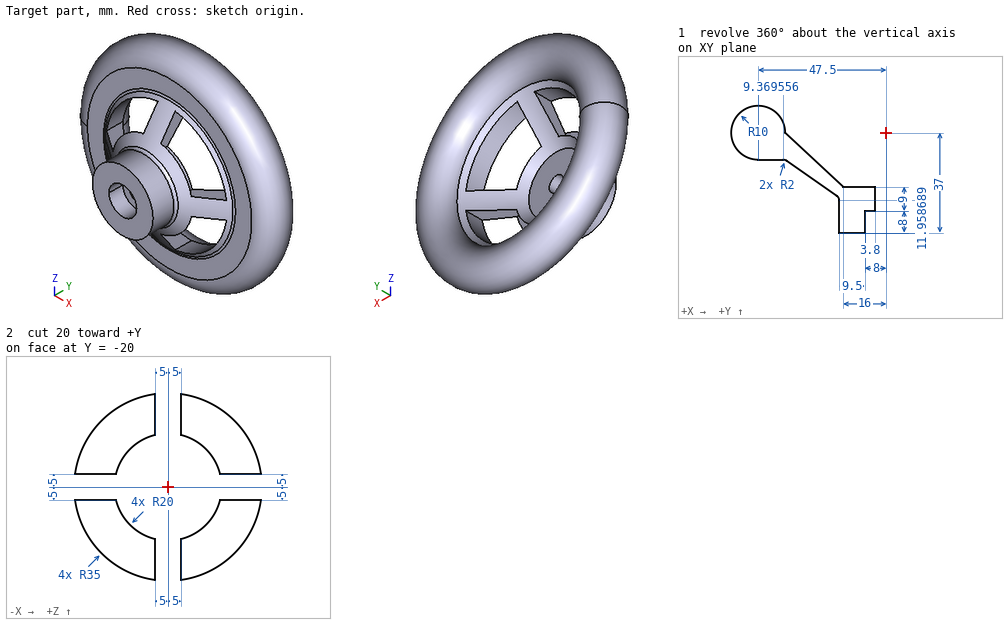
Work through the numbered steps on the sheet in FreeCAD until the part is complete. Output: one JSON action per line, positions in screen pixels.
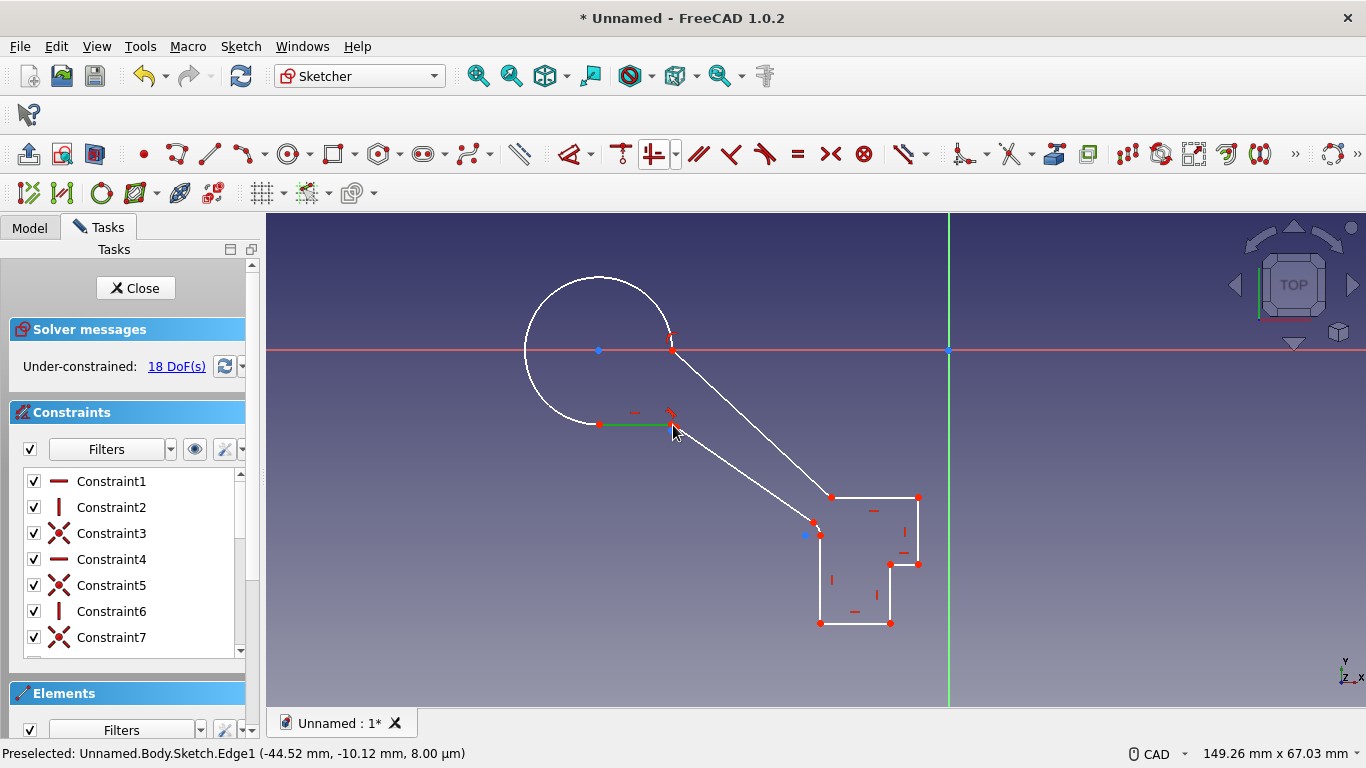
{"action": "left_click", "coordinate": [609, 278]}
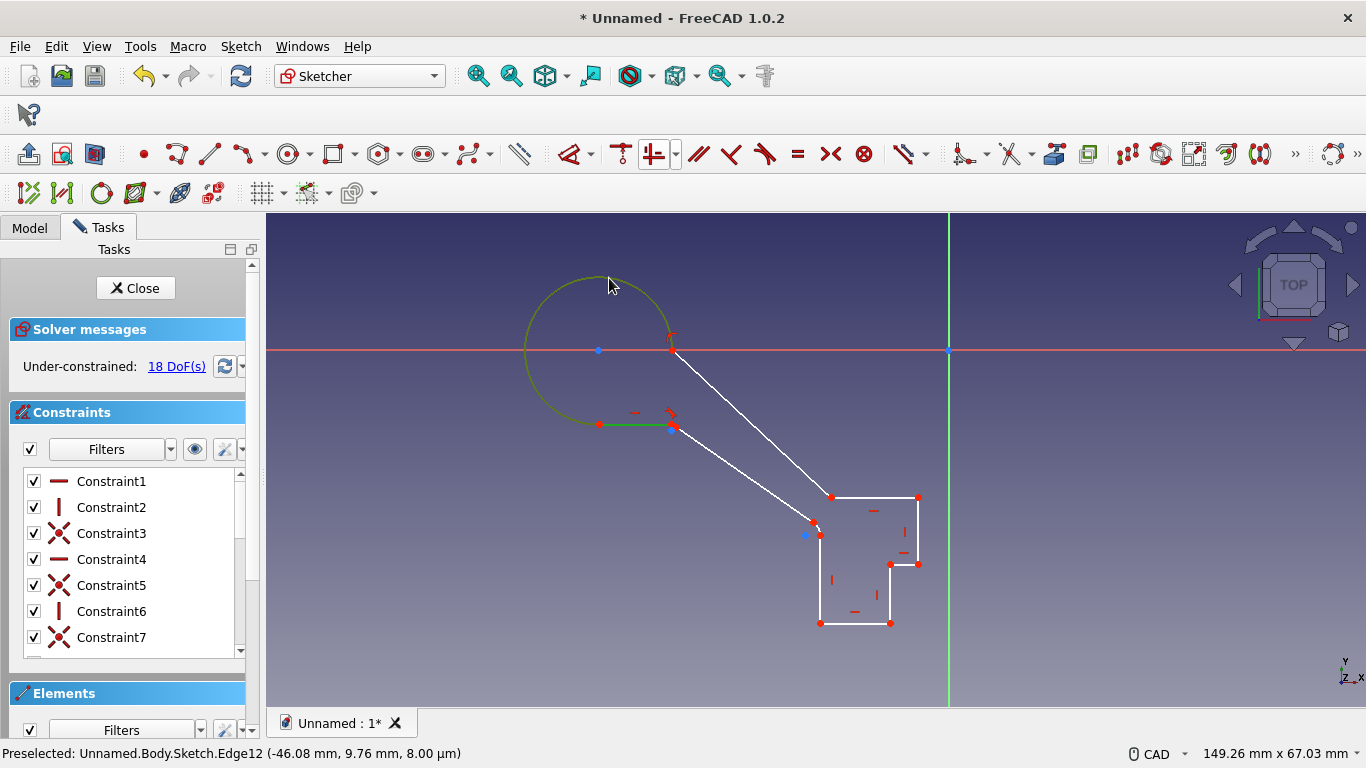
{"action": "key", "text": "t"}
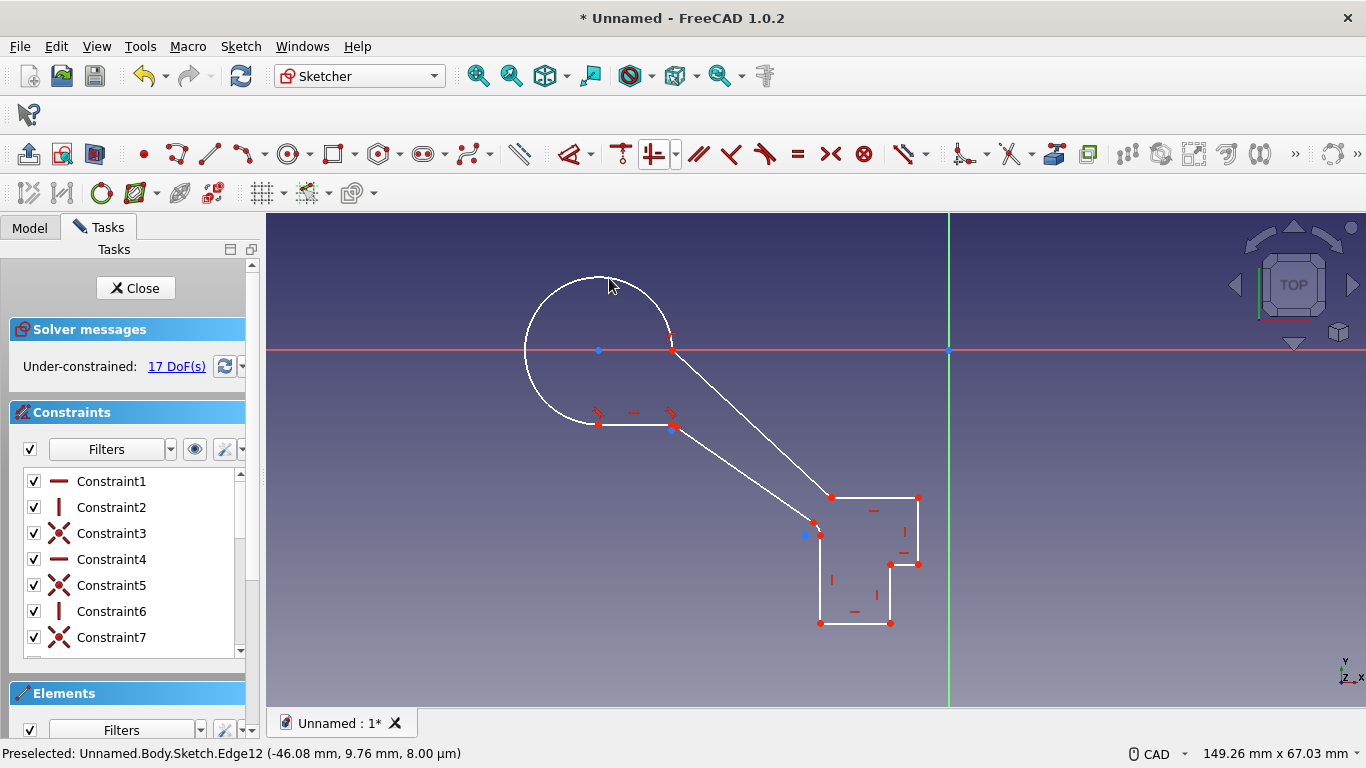
{"action": "left_click", "coordinate": [718, 456]}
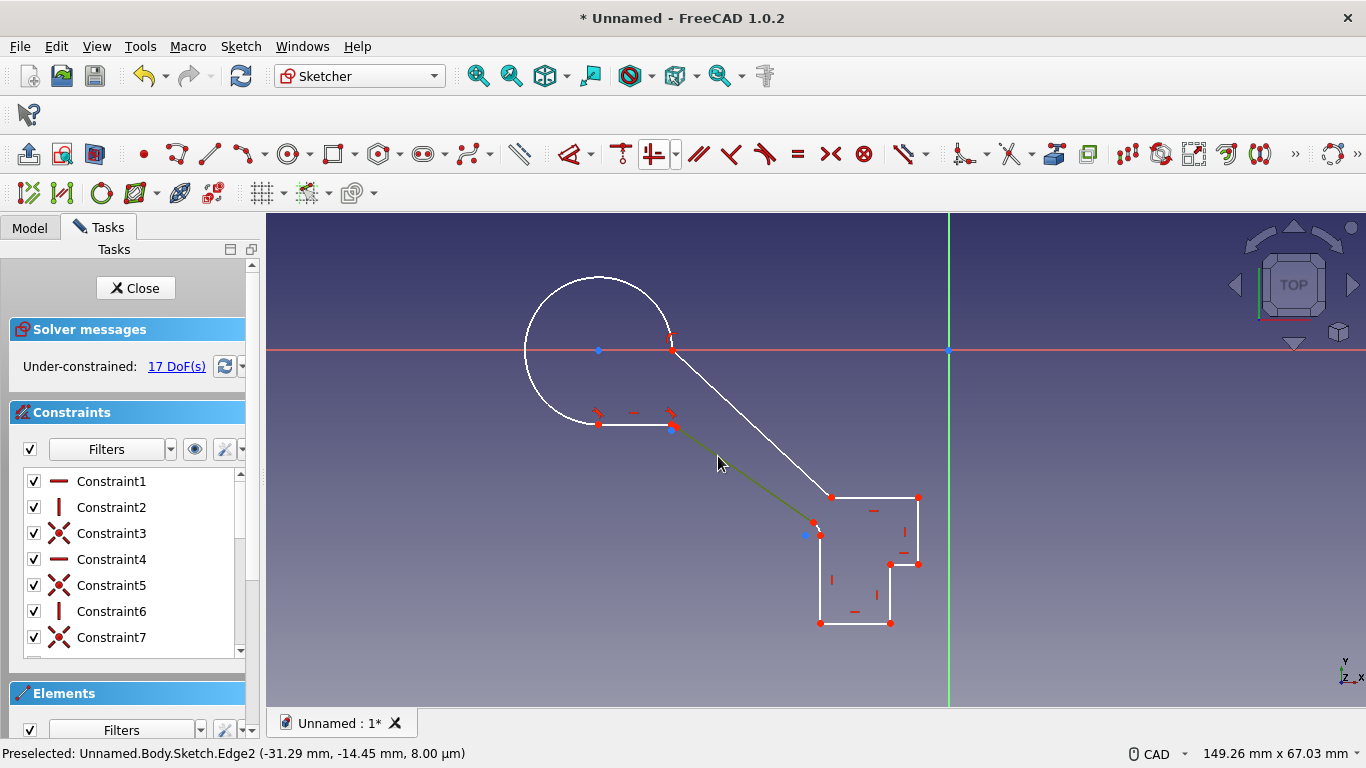
{"action": "scroll", "coordinate": [674, 425], "scroll_direction": "up", "scroll_amount": 8}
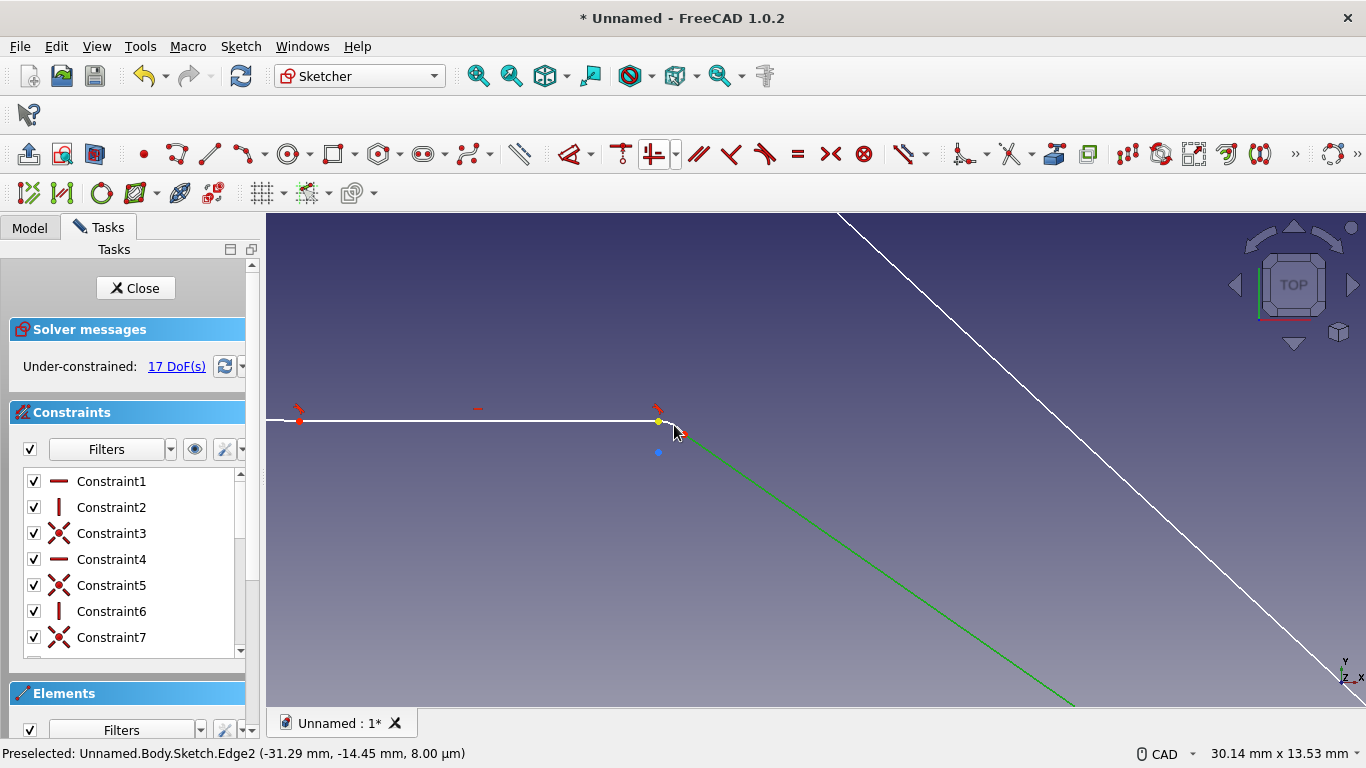
{"action": "left_click", "coordinate": [673, 425]}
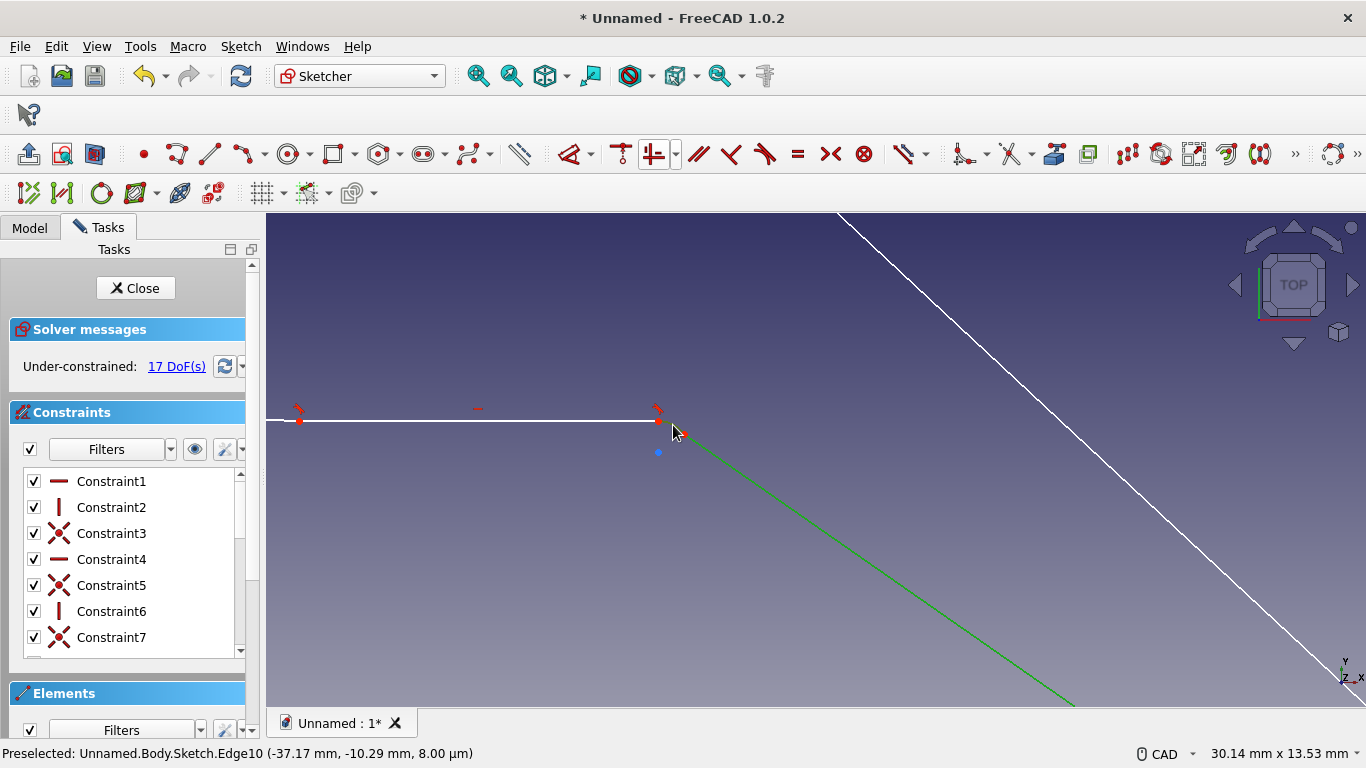
{"action": "key", "text": "t"}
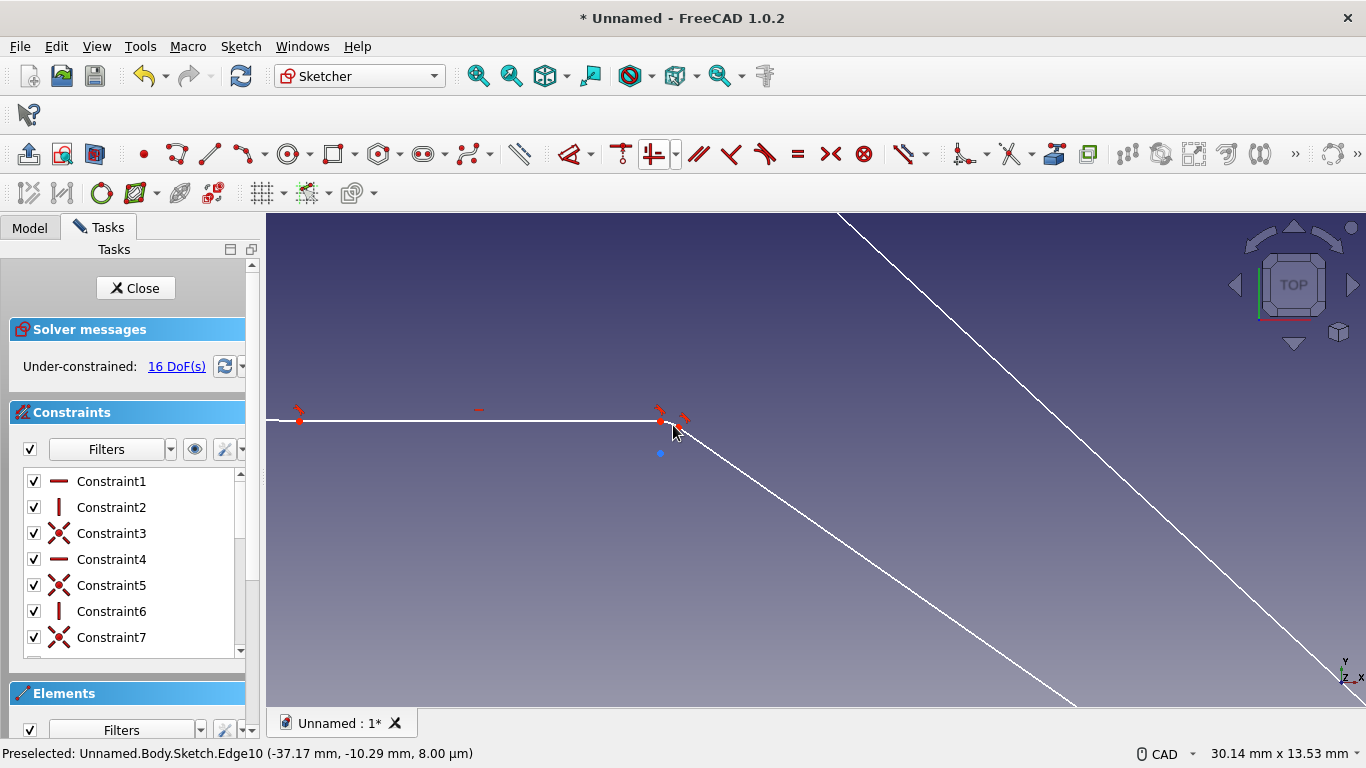
{"action": "scroll", "coordinate": [674, 425], "scroll_direction": "down", "scroll_amount": 8}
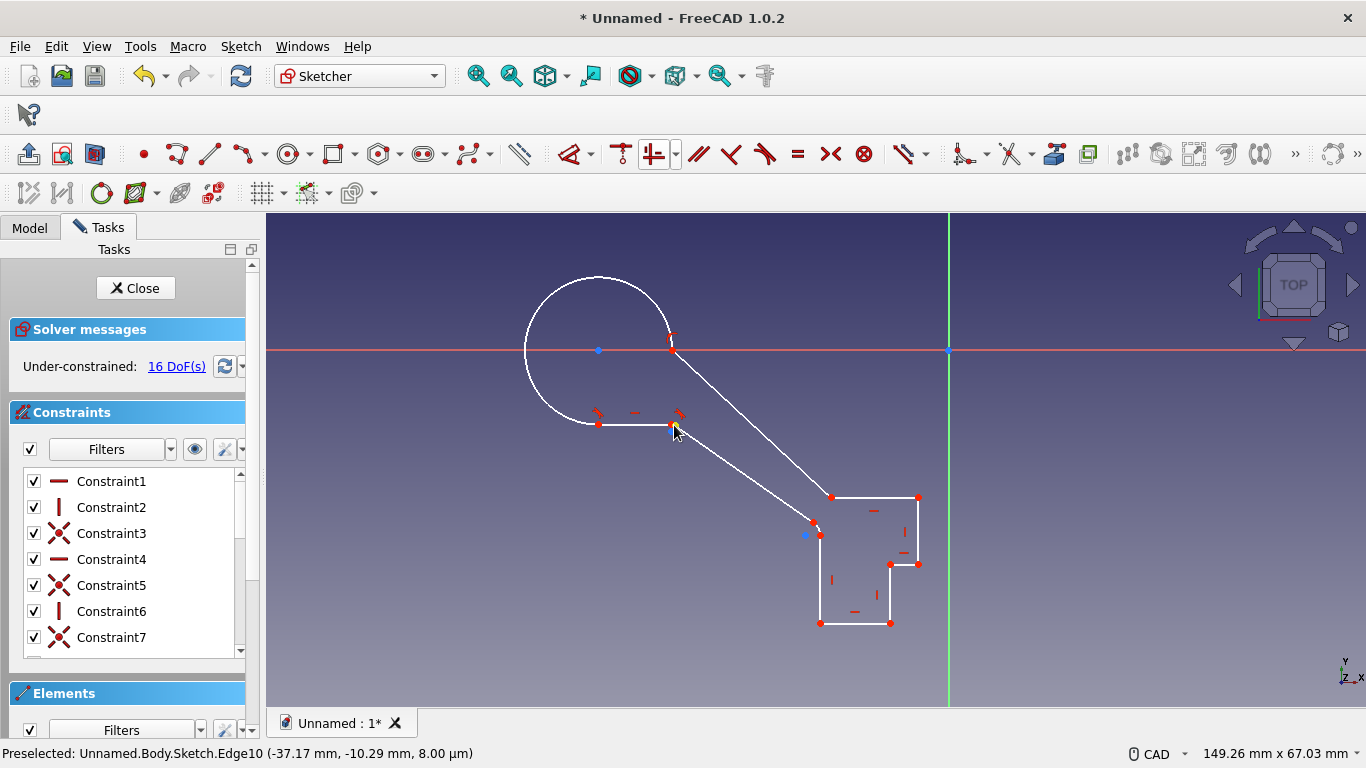
{"action": "left_click", "coordinate": [717, 455]}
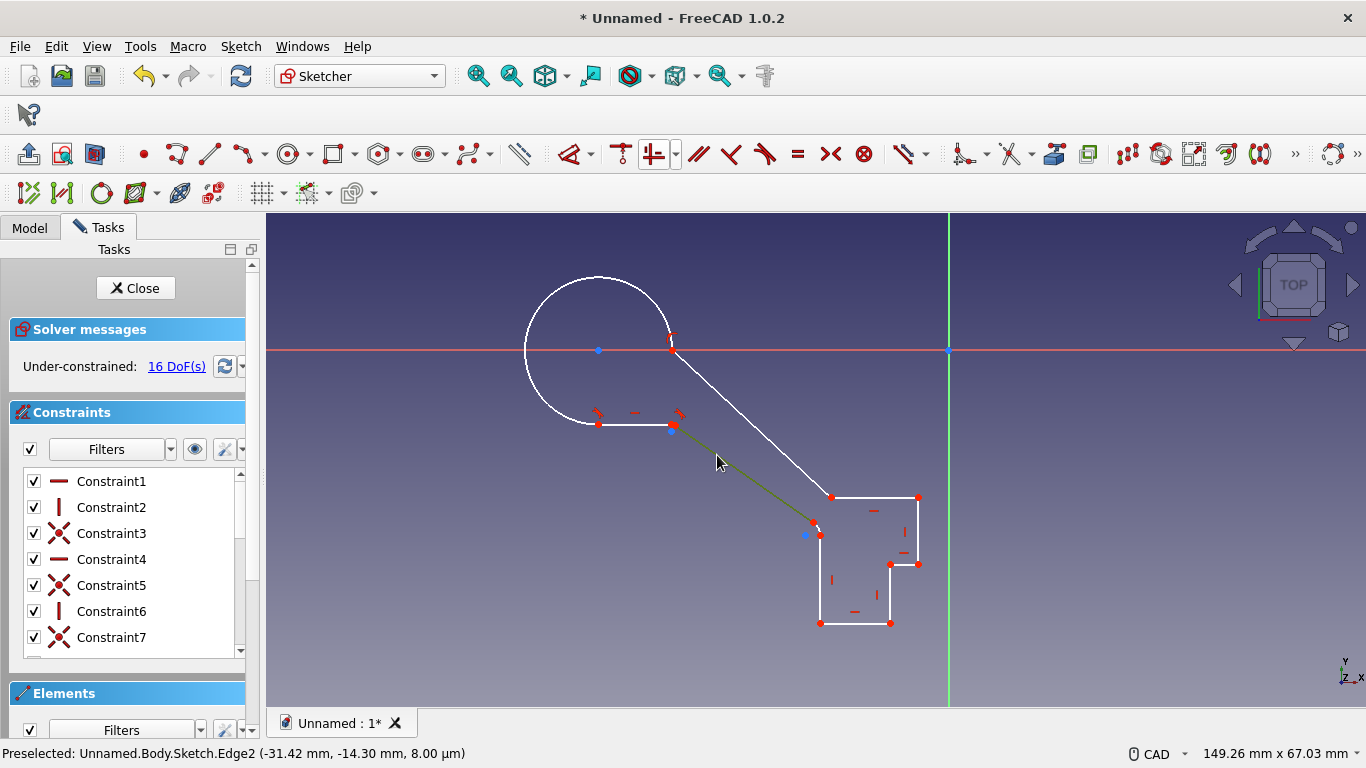
{"action": "scroll", "coordinate": [818, 528], "scroll_direction": "up", "scroll_amount": 4}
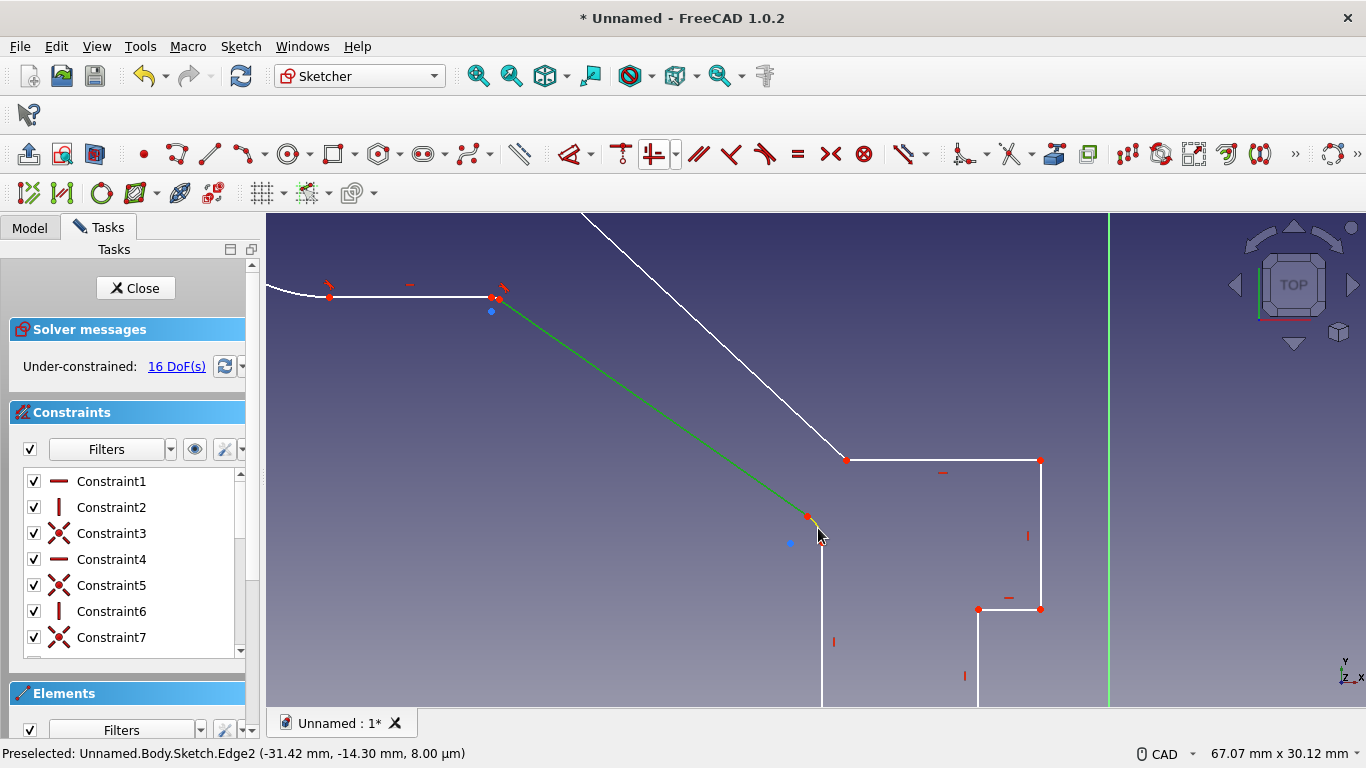
{"action": "left_click", "coordinate": [818, 528]}